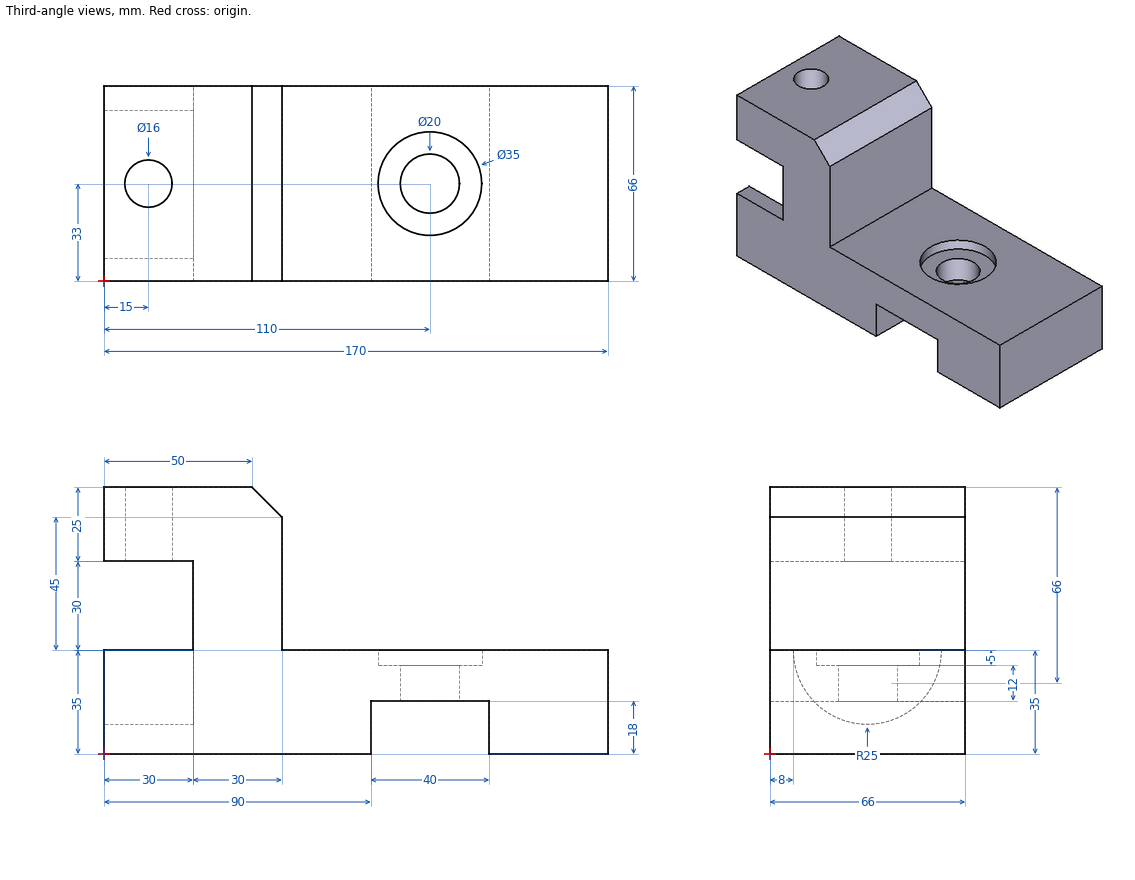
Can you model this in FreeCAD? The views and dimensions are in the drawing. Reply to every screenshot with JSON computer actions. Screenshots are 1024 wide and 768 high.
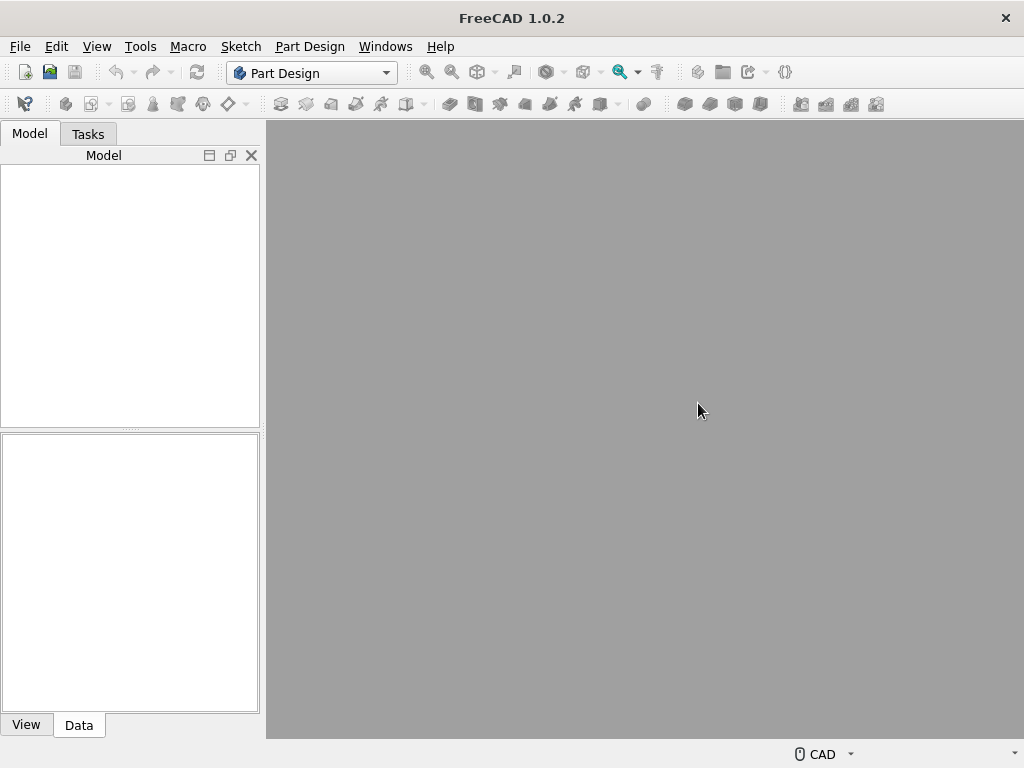
{"action": "left_click", "coordinate": [25, 72]}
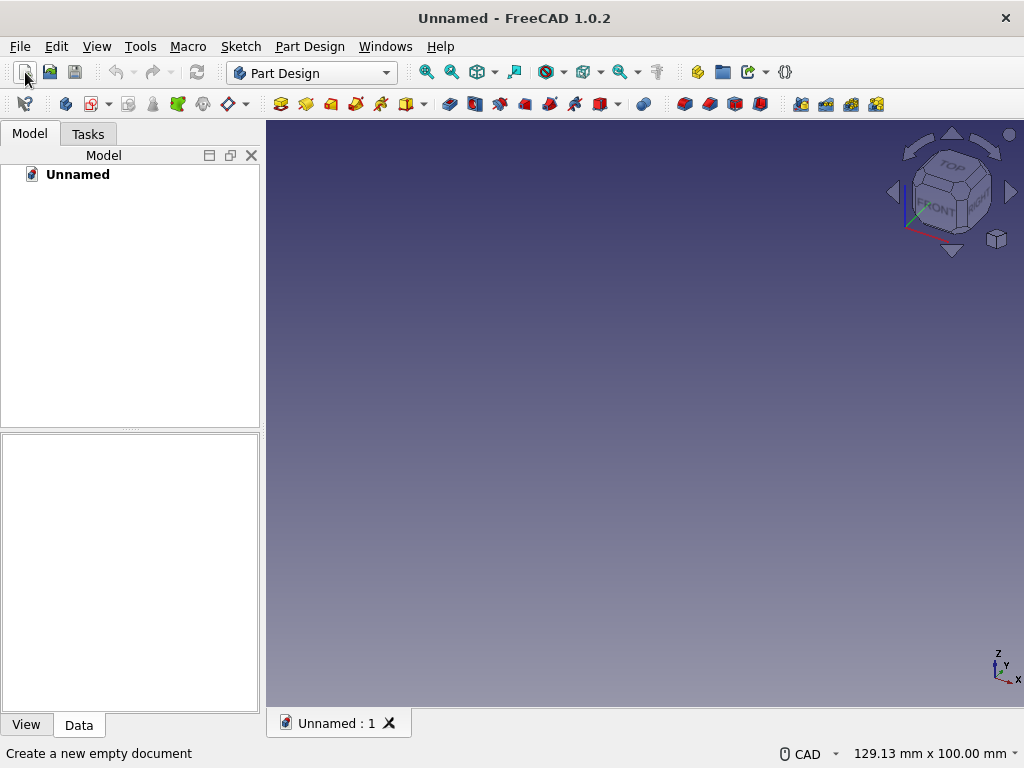
{"action": "left_click", "coordinate": [90, 104]}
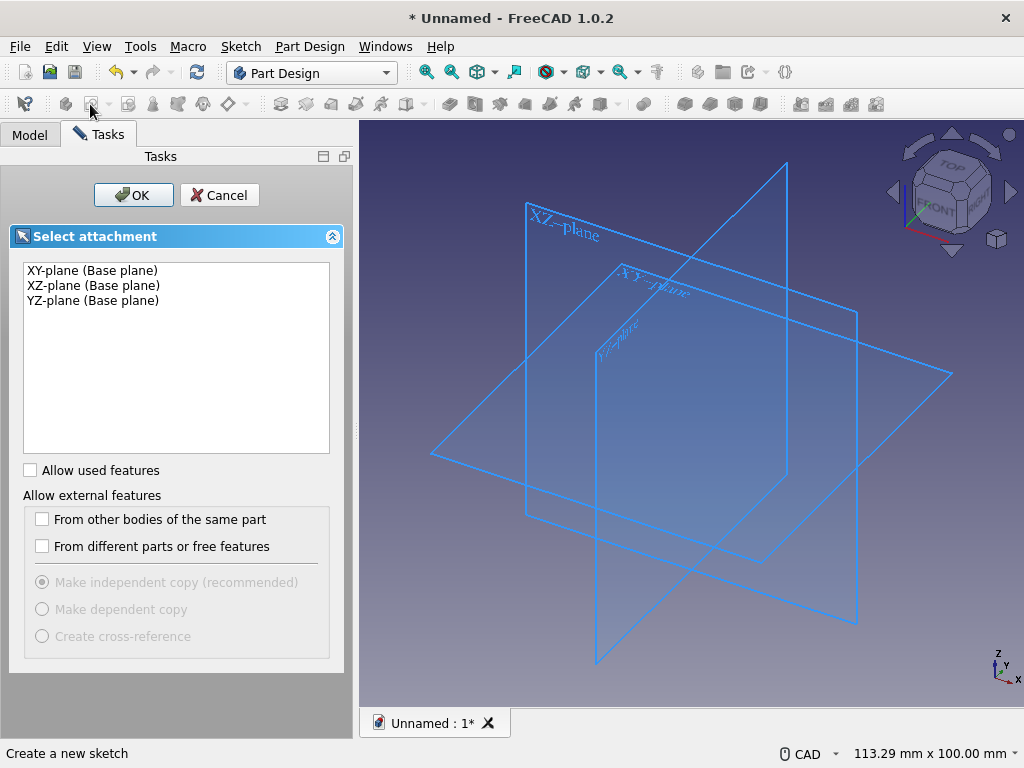
{"action": "left_click", "coordinate": [84, 270]}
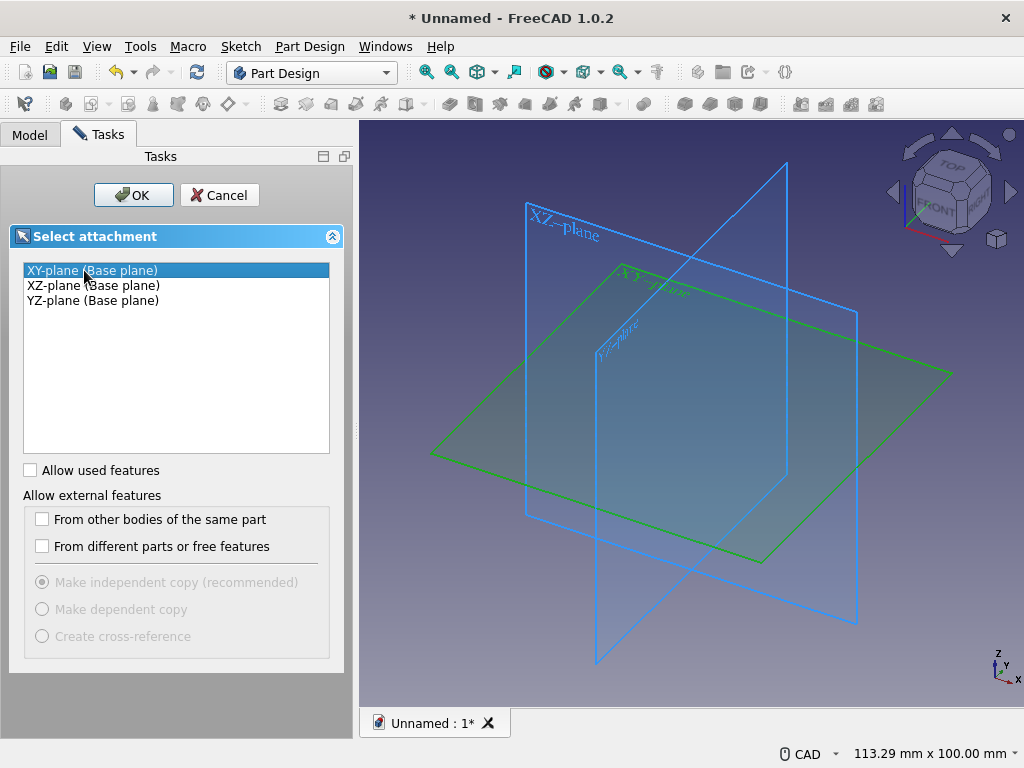
{"action": "left_click", "coordinate": [134, 195]}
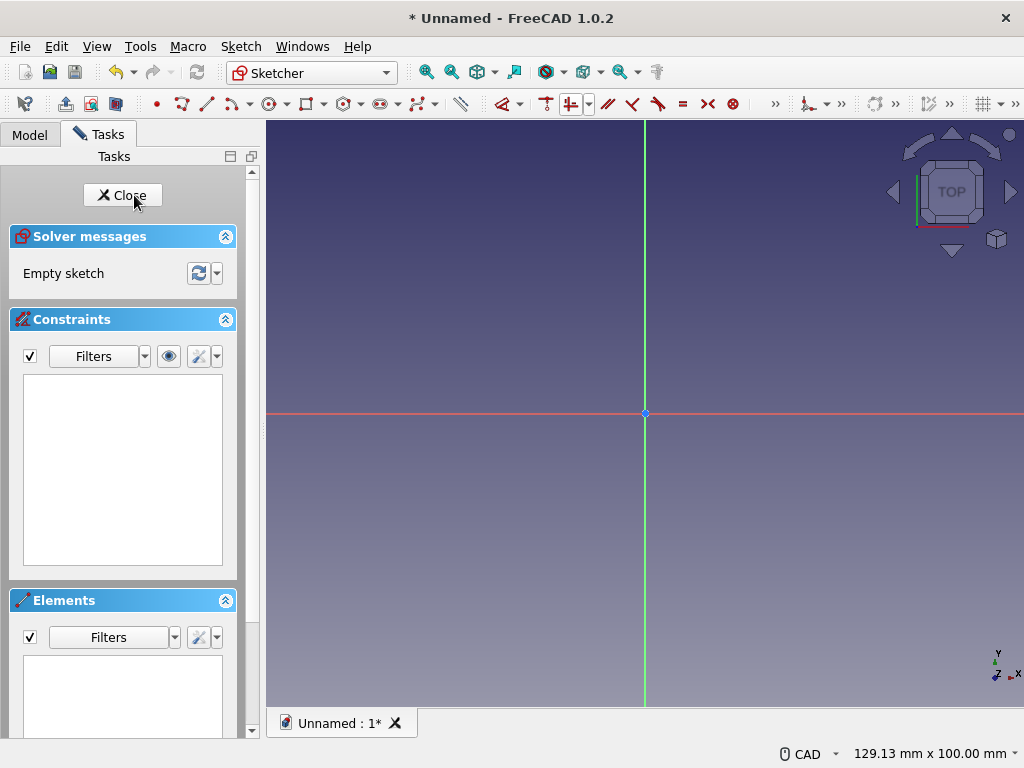
{"action": "scroll", "coordinate": [294, 526], "scroll_direction": "down", "scroll_amount": 5}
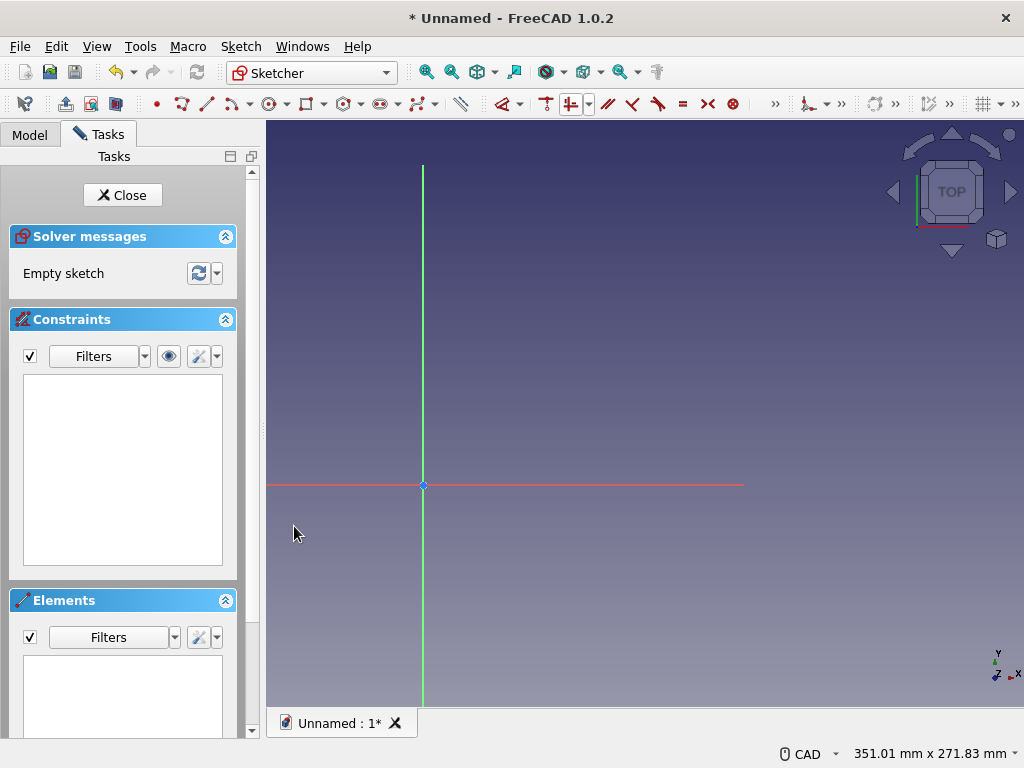
{"action": "key", "text": "g r"}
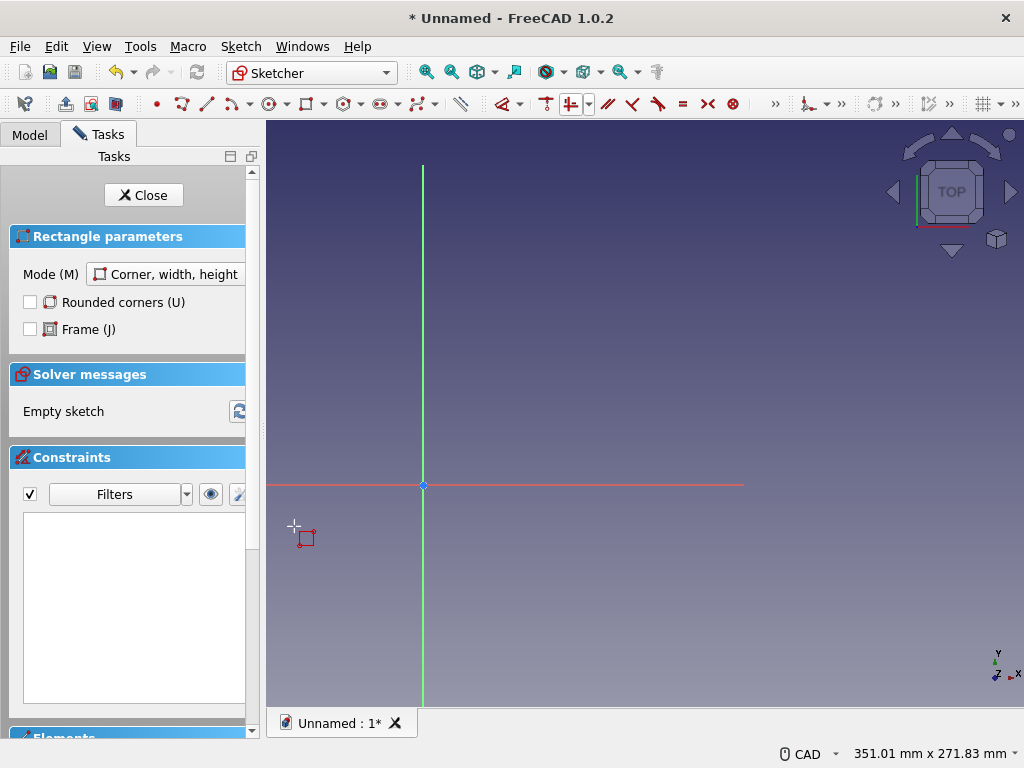
{"action": "left_click", "coordinate": [423, 485]}
{"action": "mouse_move", "coordinate": [790, 343]}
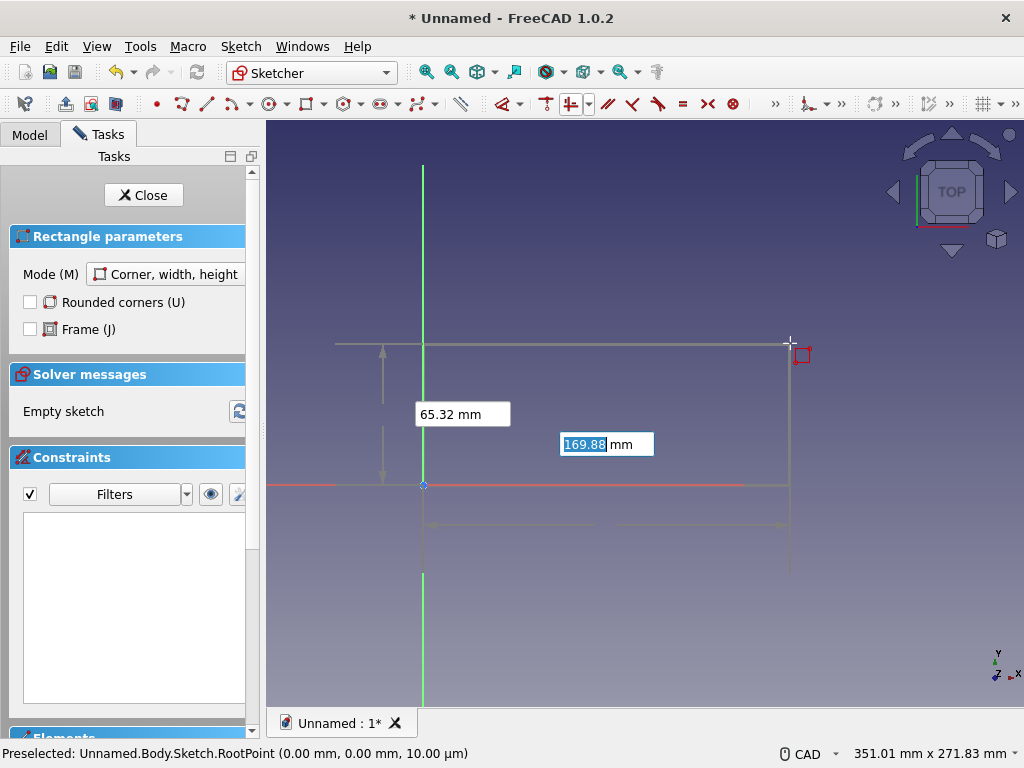
{"action": "type", "text": "170"}
{"action": "key", "text": "Tab"}
{"action": "type", "text": "66"}
{"action": "key", "text": "Return"}
{"action": "key", "text": "Escape"}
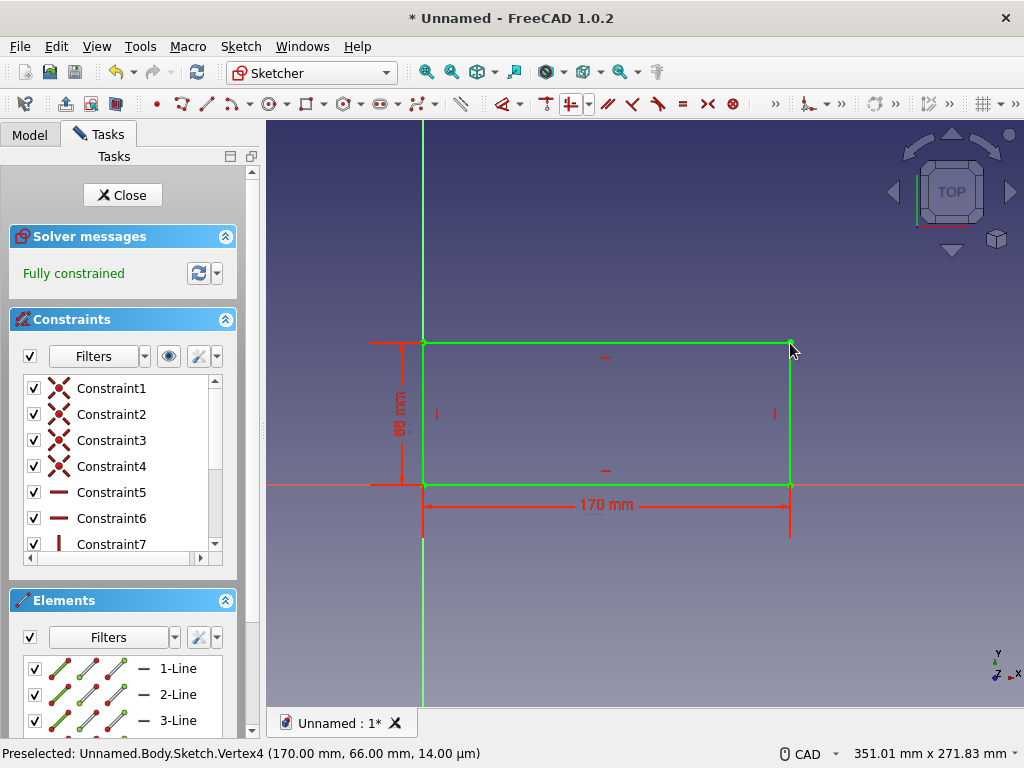
{"action": "left_click", "coordinate": [123, 195]}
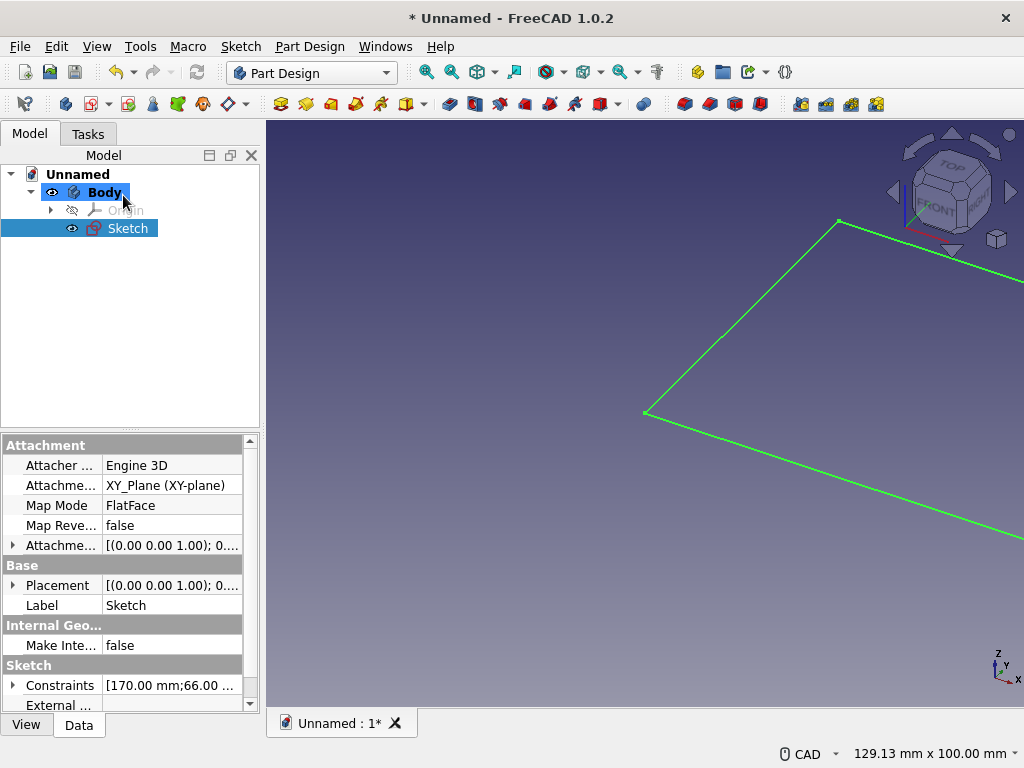
{"action": "left_click", "coordinate": [281, 104]}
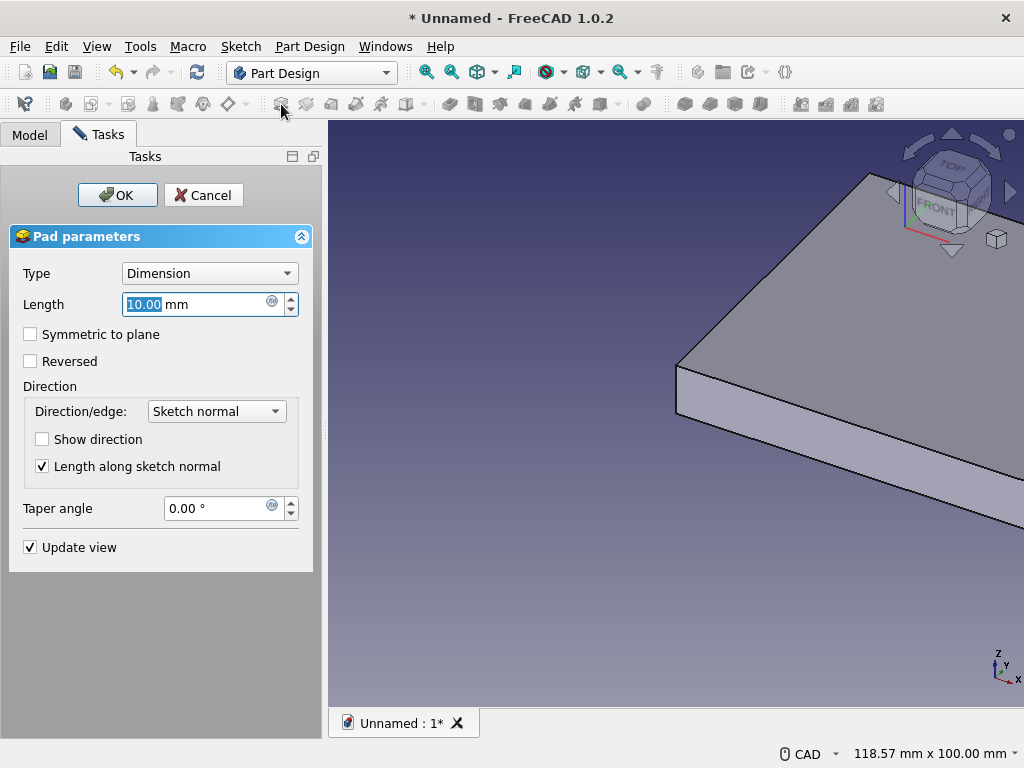
{"action": "type", "text": "35"}
{"action": "key", "text": "Tab"}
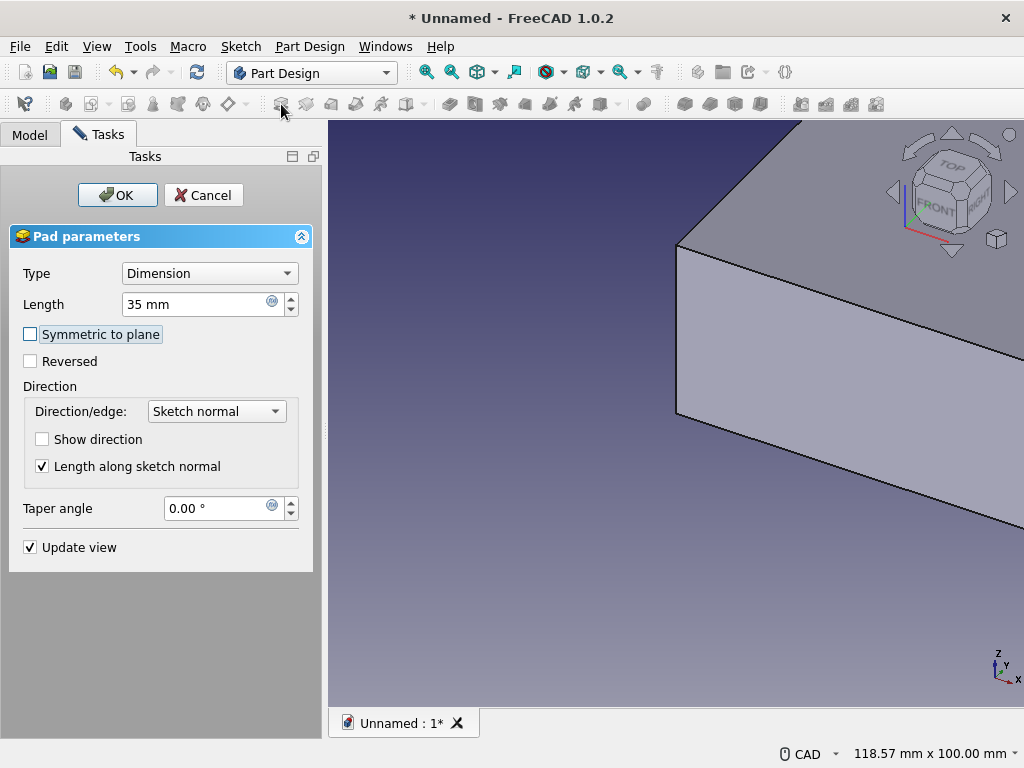
{"action": "left_click", "coordinate": [118, 195]}